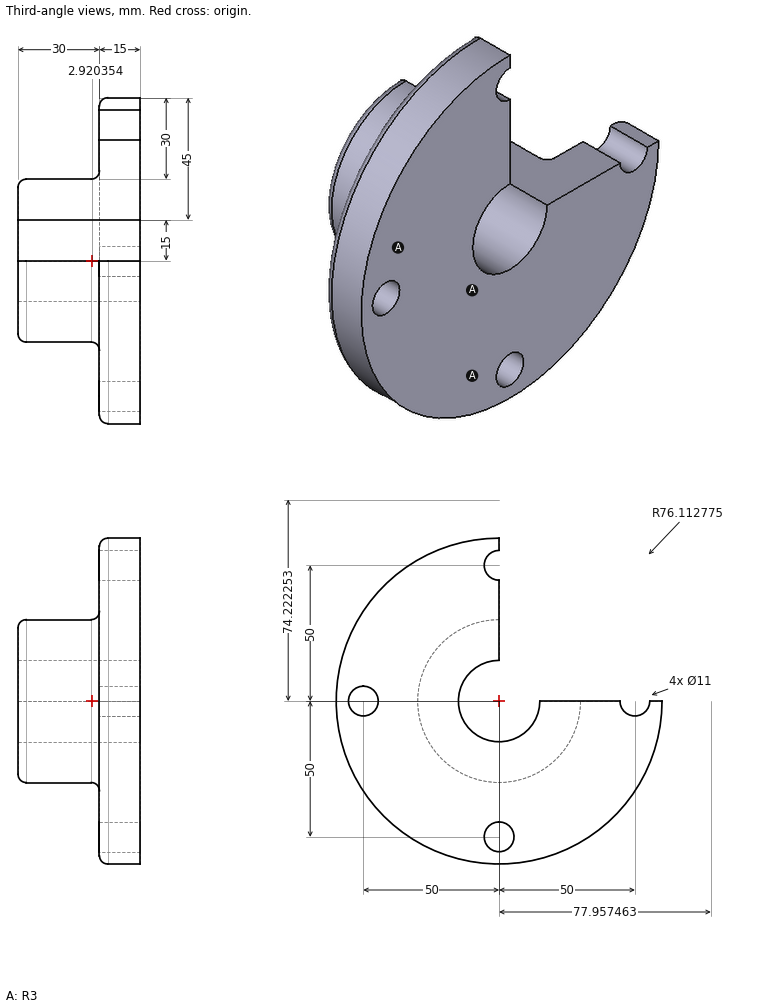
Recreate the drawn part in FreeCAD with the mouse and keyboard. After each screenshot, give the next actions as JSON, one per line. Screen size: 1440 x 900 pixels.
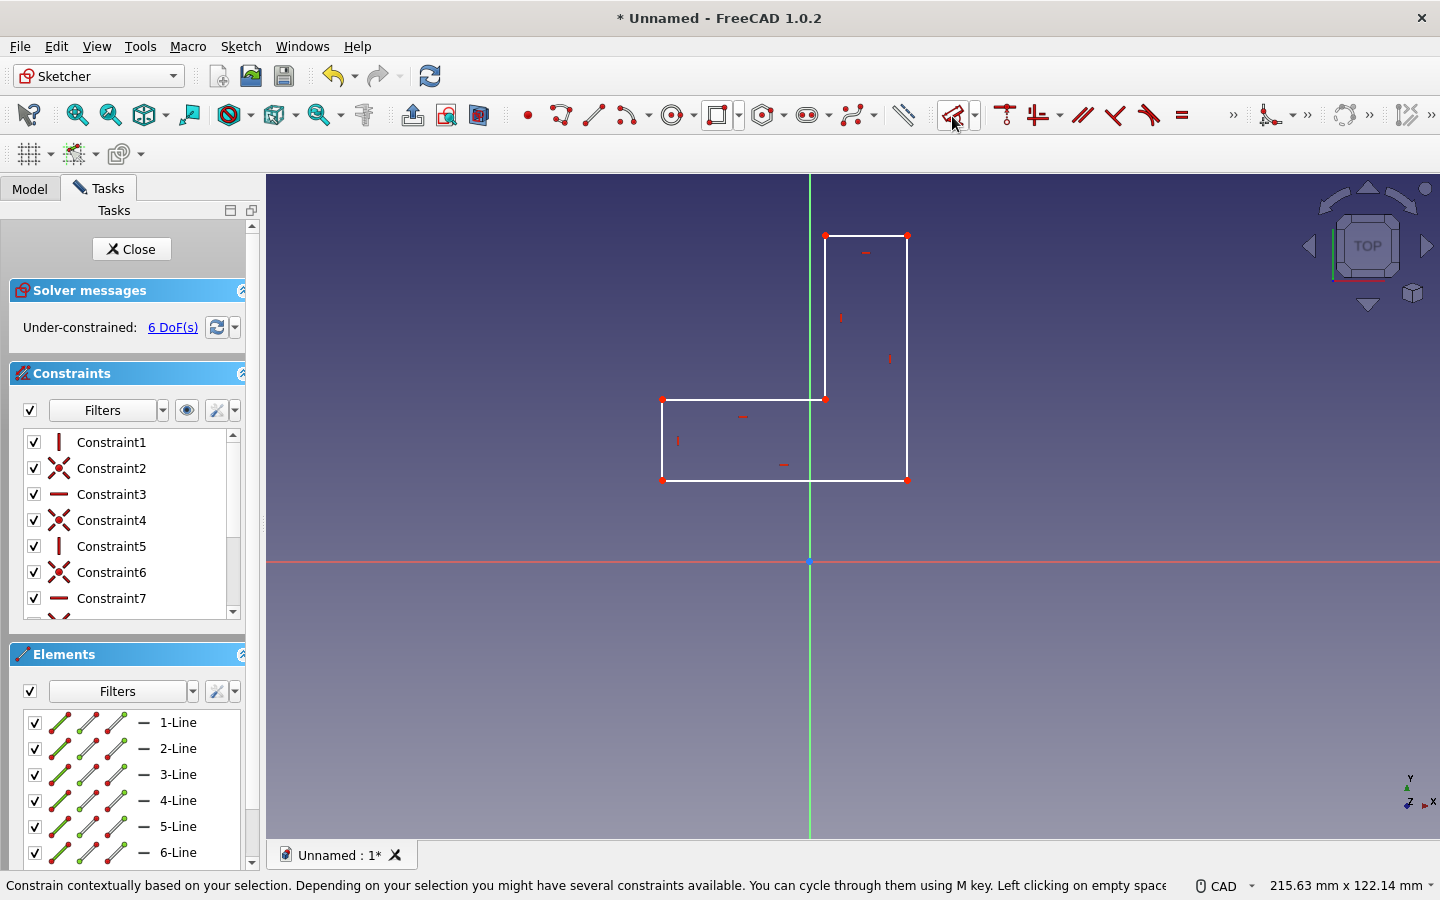
{"action": "left_click", "coordinate": [907, 407]}
{"action": "left_click", "coordinate": [941, 359]}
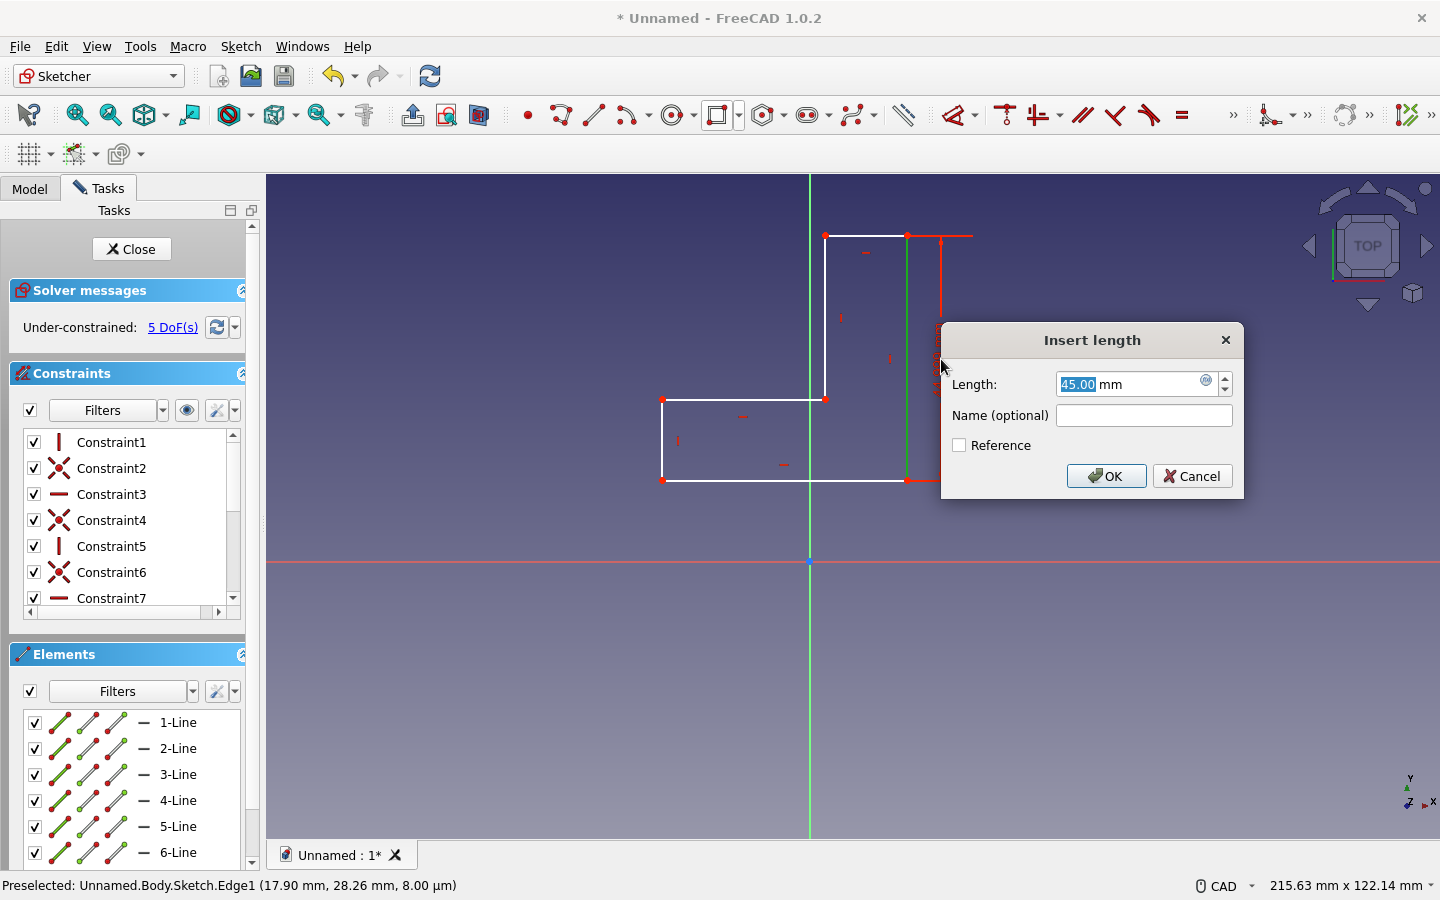
{"action": "type", "text": "45"}
{"action": "key", "text": "Return"}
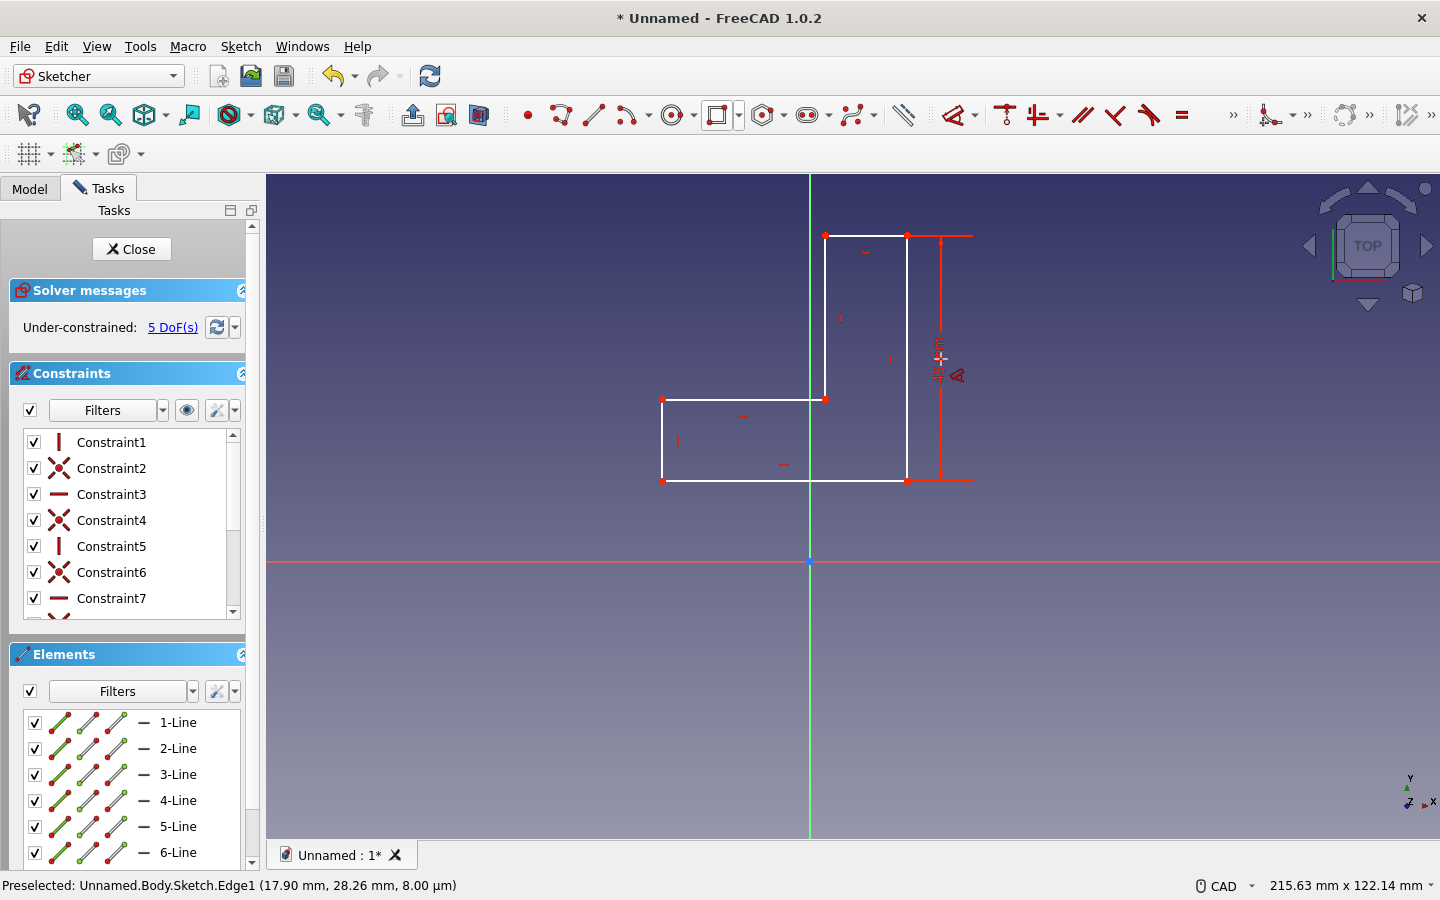
{"action": "left_click", "coordinate": [882, 236]}
{"action": "left_click", "coordinate": [866, 202]}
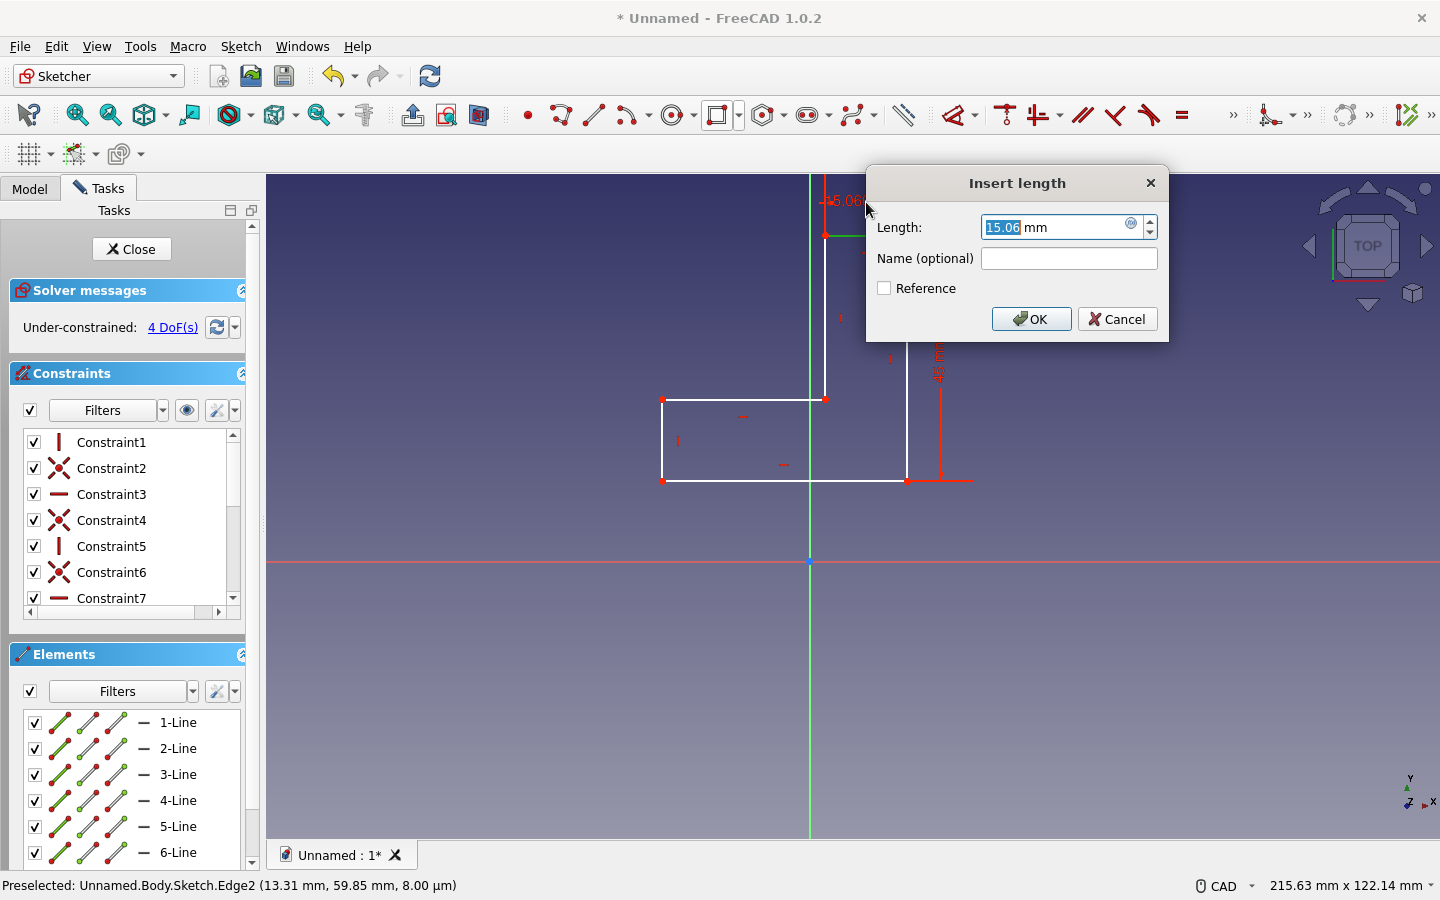
{"action": "type", "text": "15"}
{"action": "key", "text": "Return"}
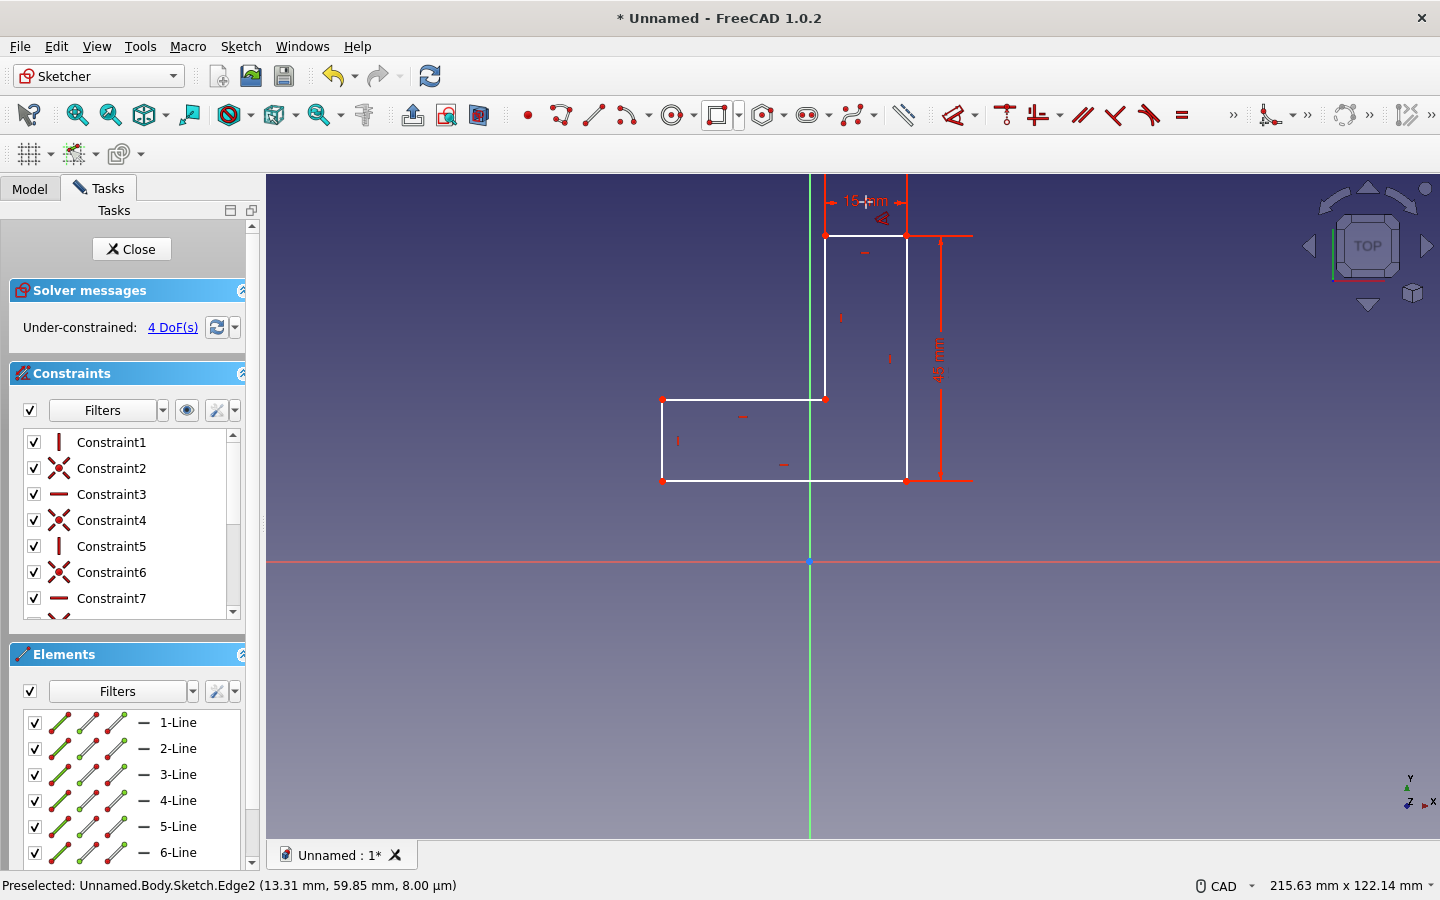
{"action": "left_click", "coordinate": [825, 285]}
{"action": "left_click", "coordinate": [859, 318]}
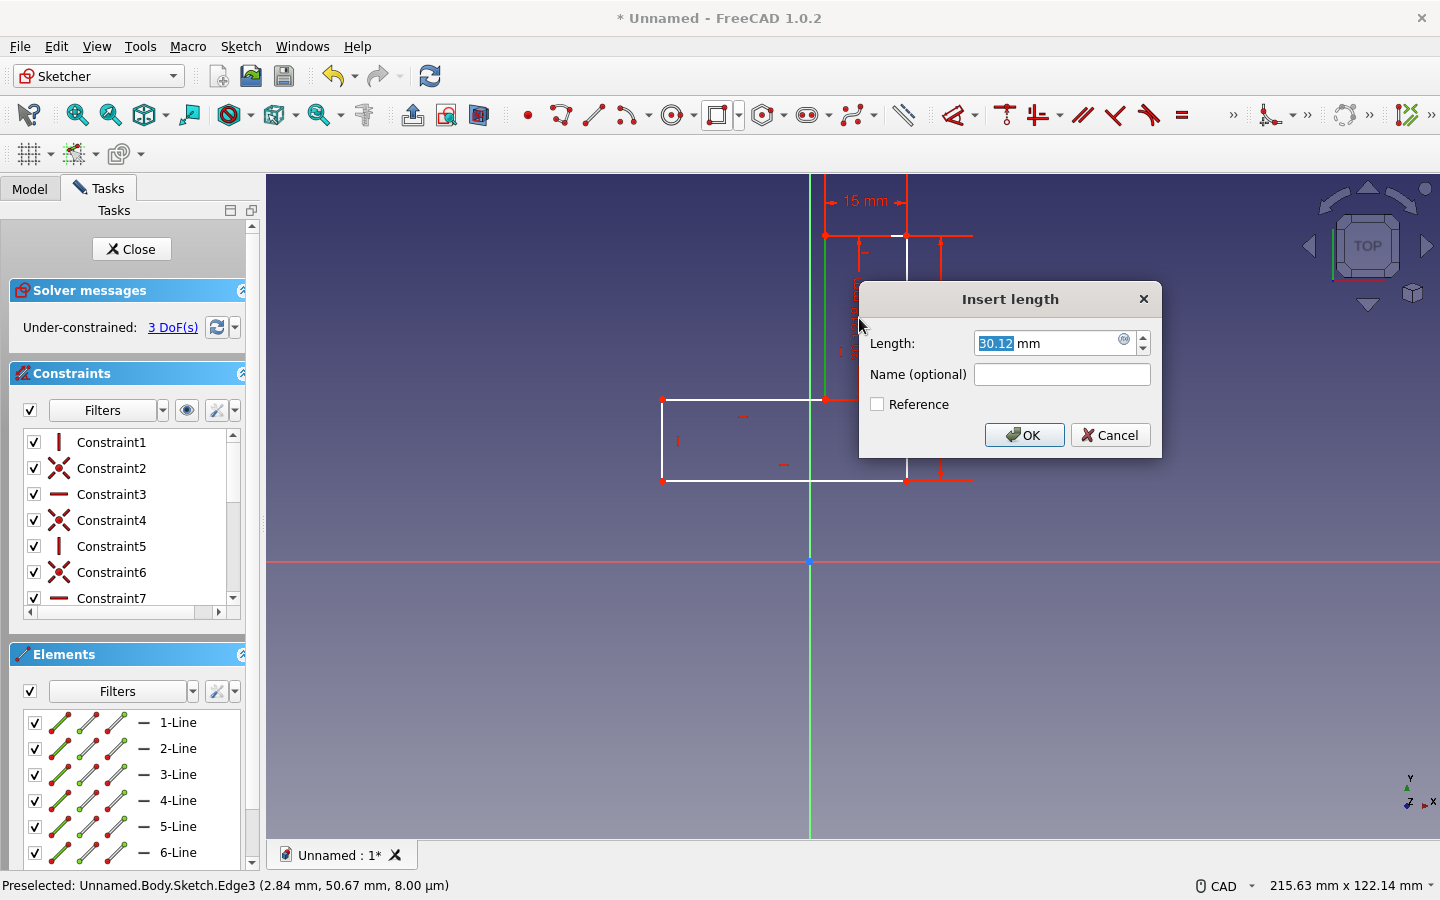
{"action": "type", "text": "30"}
{"action": "key", "text": "Return"}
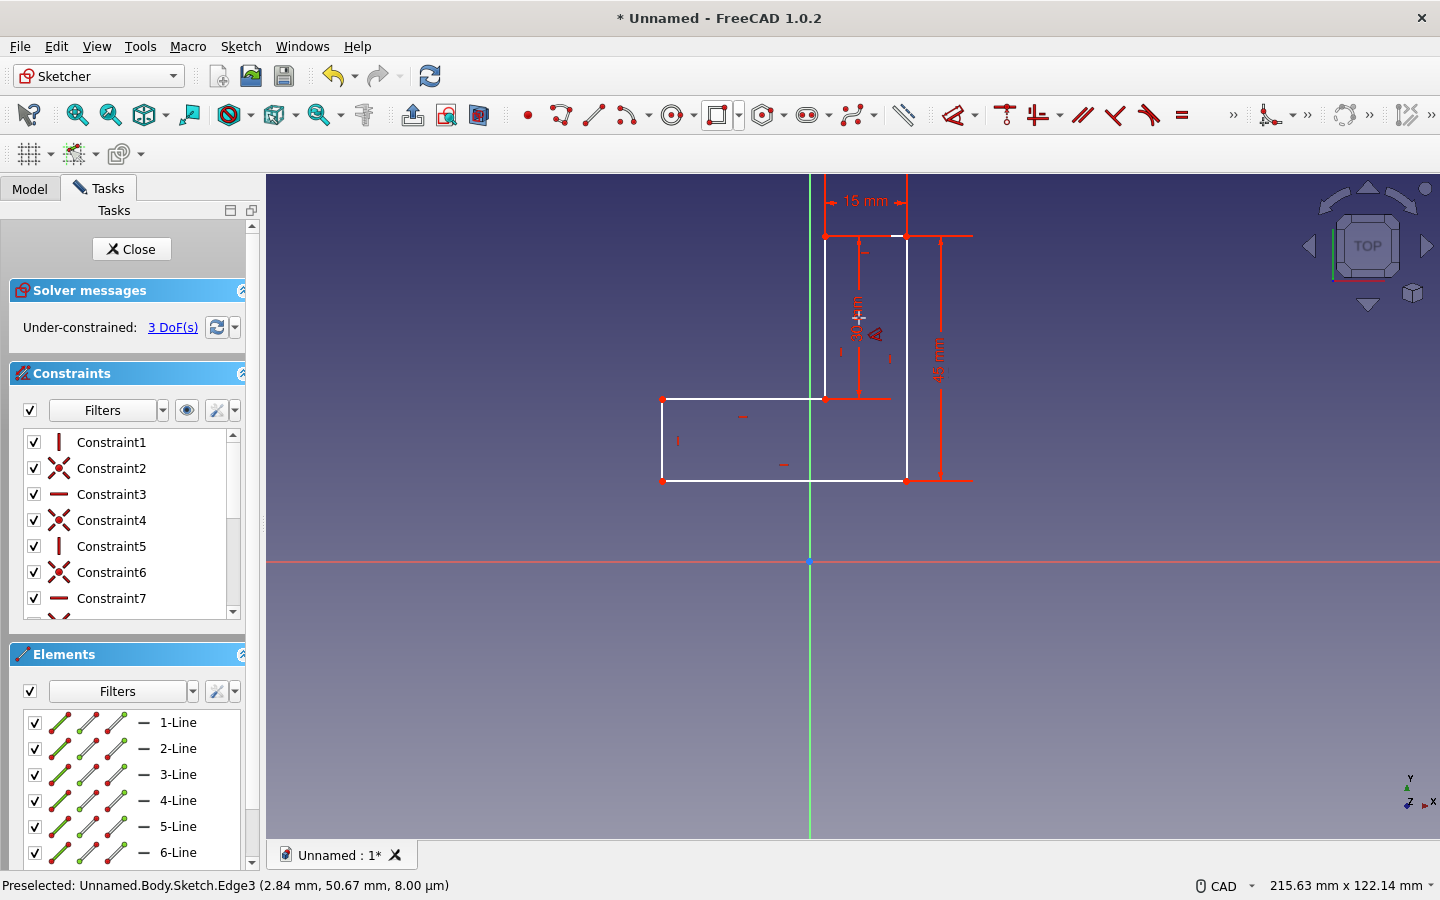
{"action": "left_click", "coordinate": [776, 399]}
{"action": "left_click", "coordinate": [744, 433]}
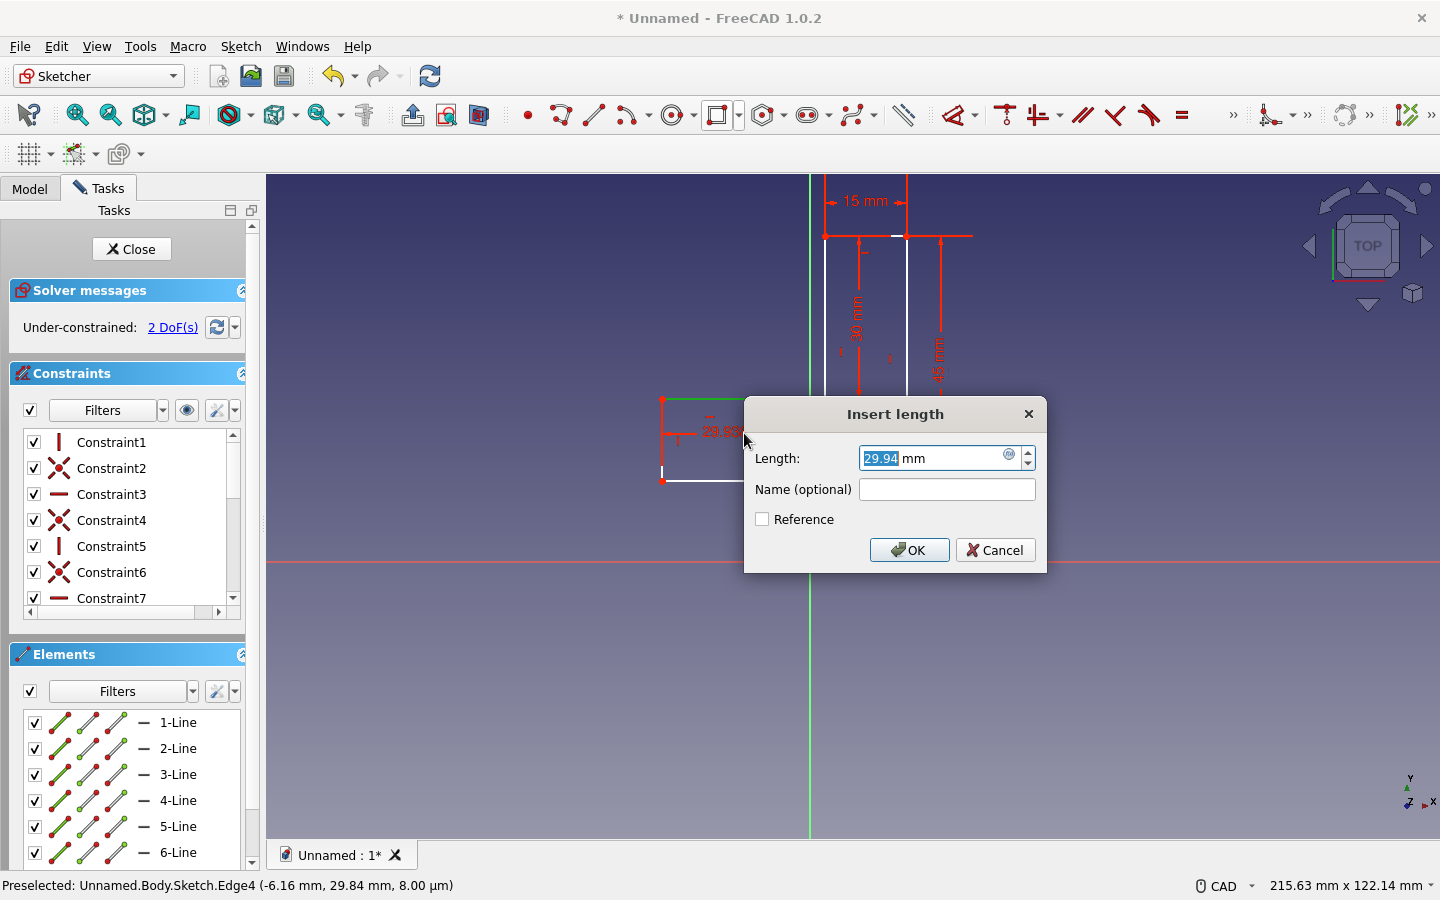
{"action": "type", "text": "30"}
{"action": "key", "text": "Return"}